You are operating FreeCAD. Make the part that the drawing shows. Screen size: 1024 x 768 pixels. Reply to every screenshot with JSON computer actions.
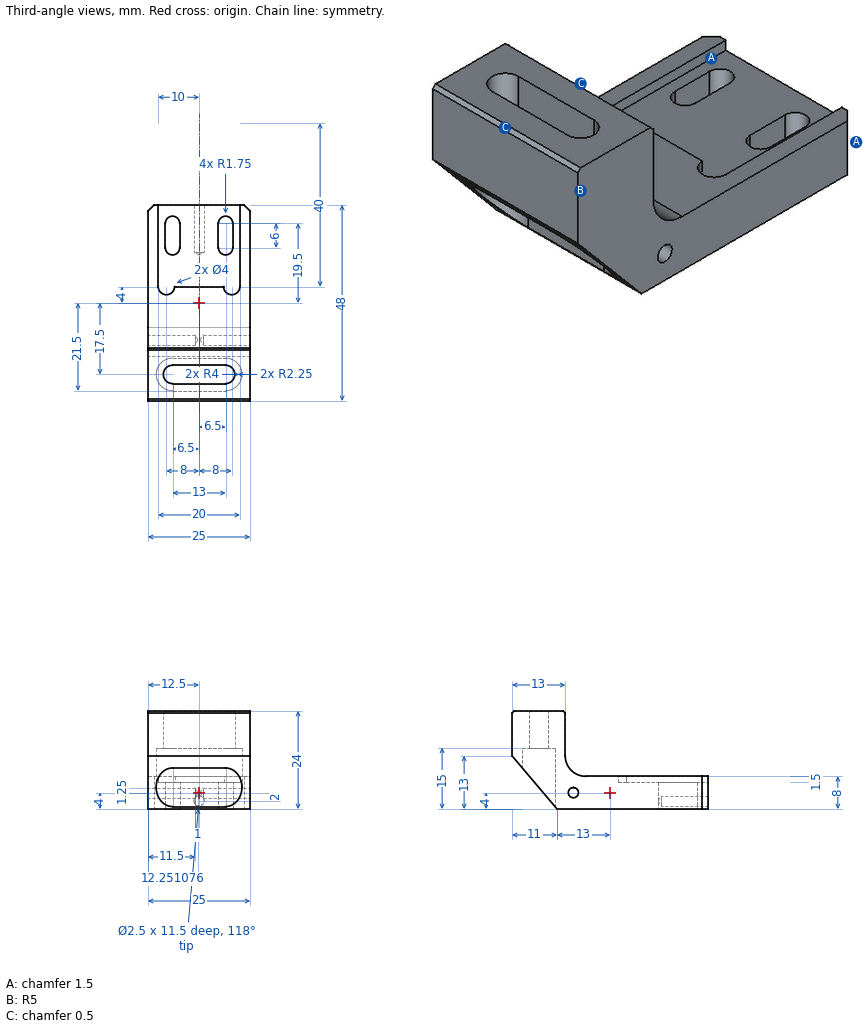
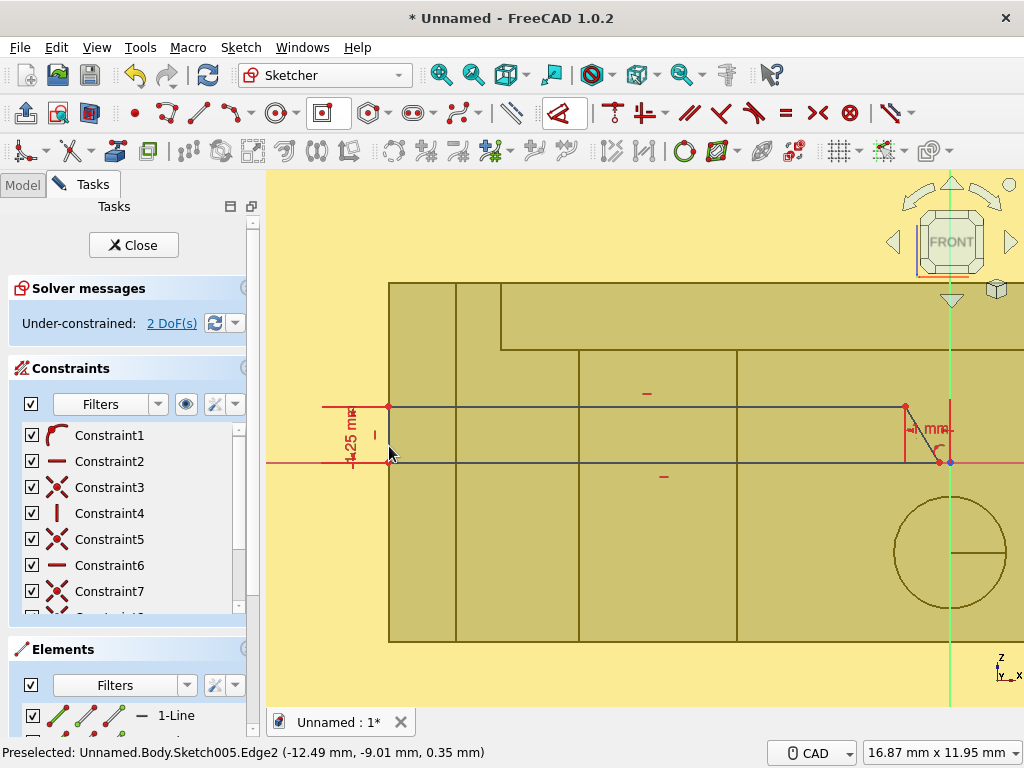
{"action": "left_click", "coordinate": [544, 407]}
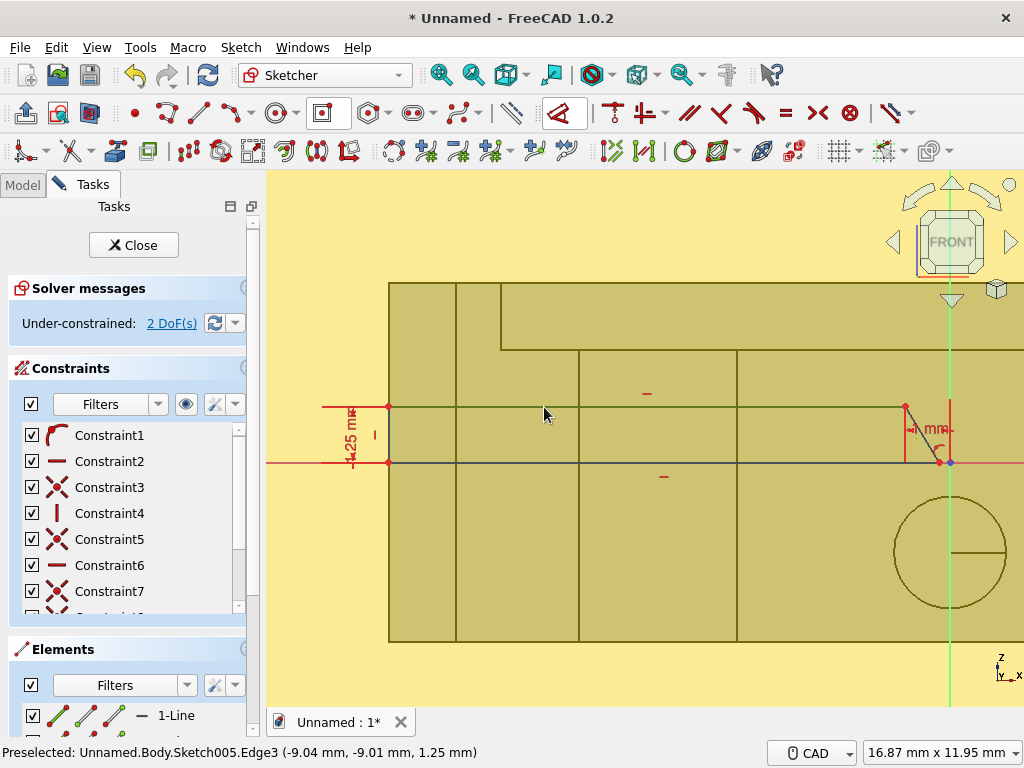
{"action": "left_click", "coordinate": [582, 114]}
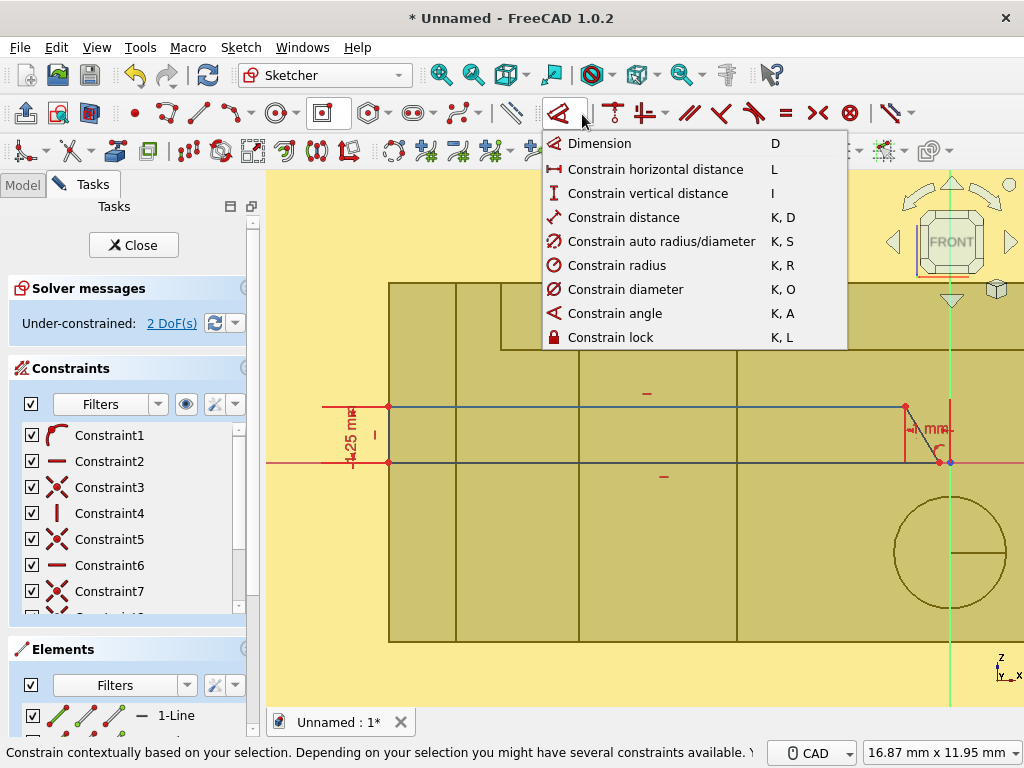
{"action": "left_click", "coordinate": [695, 169]}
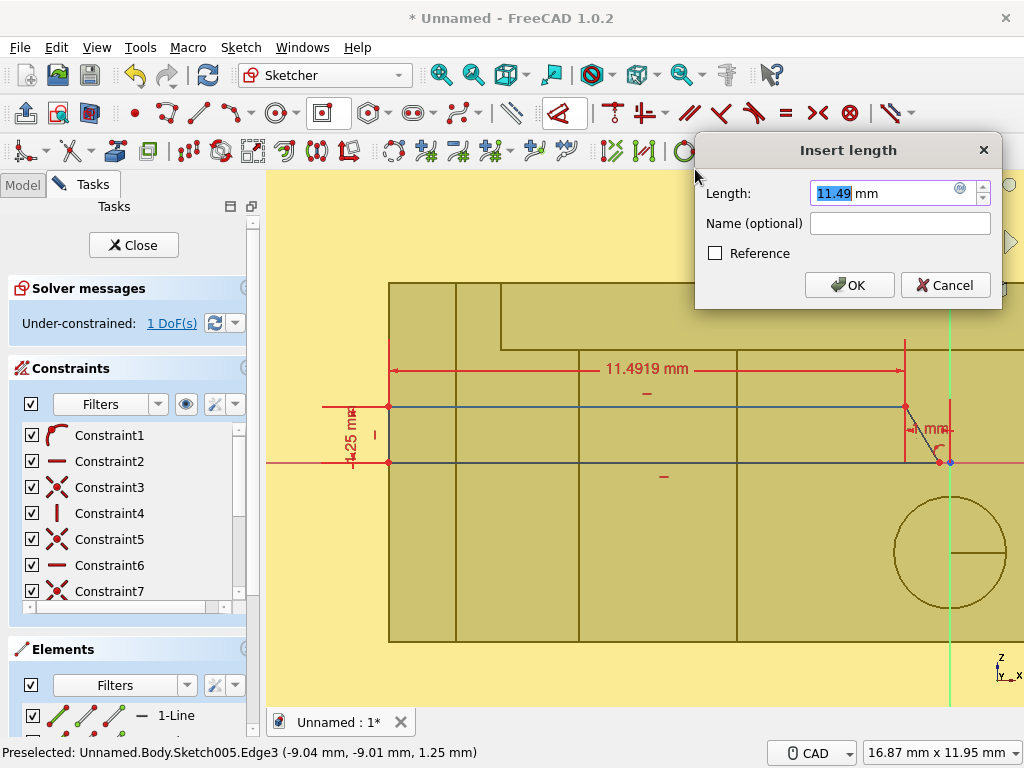
{"action": "type", "text": "11.5"}
{"action": "key", "text": "Return"}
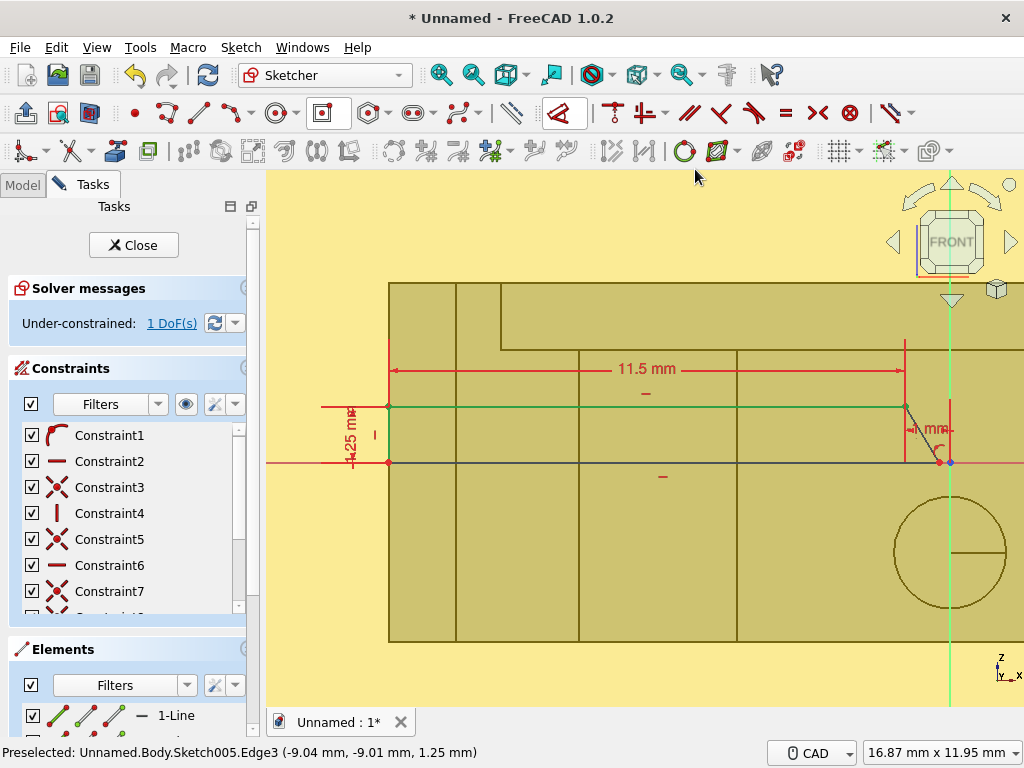
{"action": "left_click", "coordinate": [774, 463]}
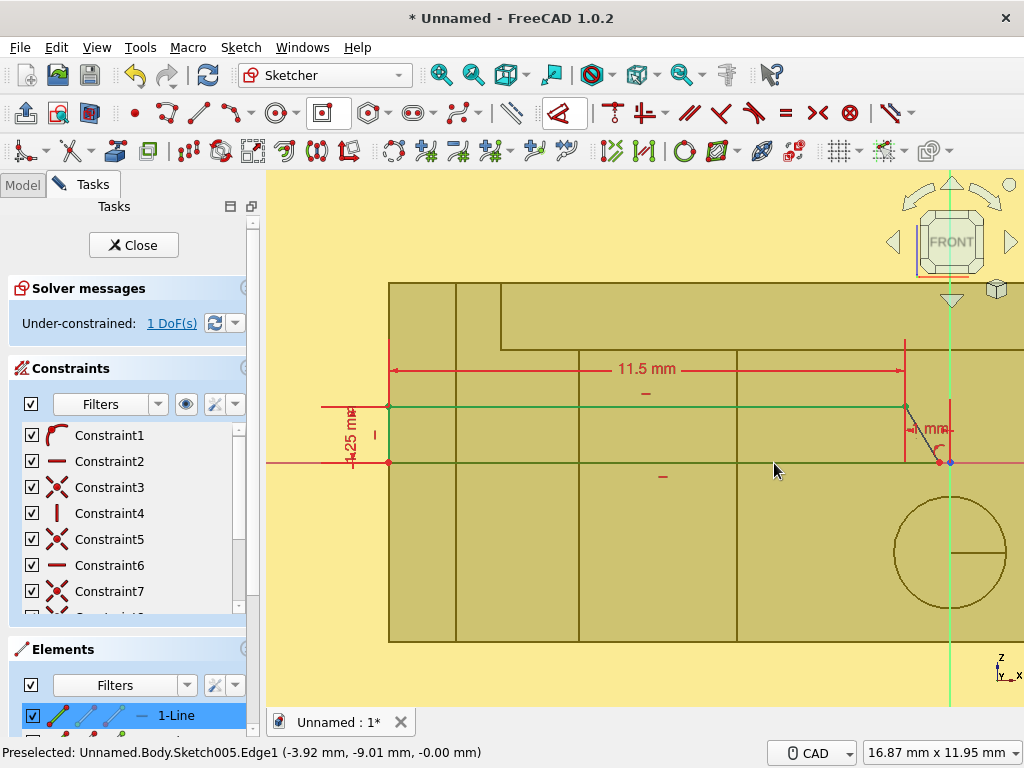
{"action": "left_click", "coordinate": [582, 114]}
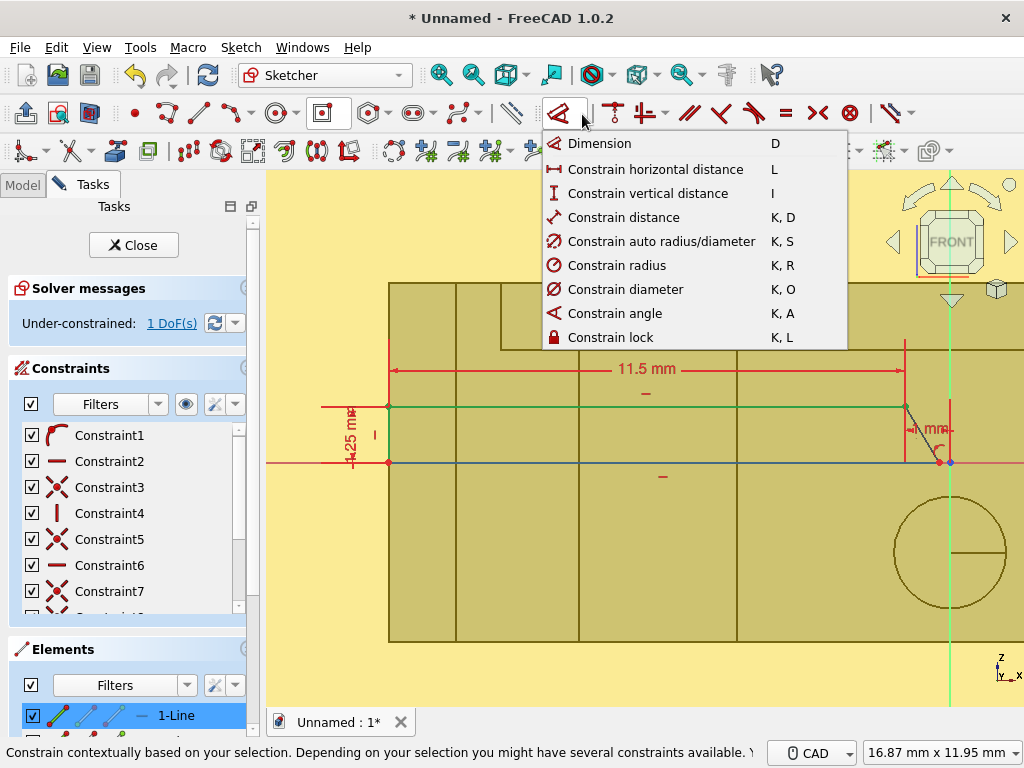
{"action": "left_click", "coordinate": [695, 169]}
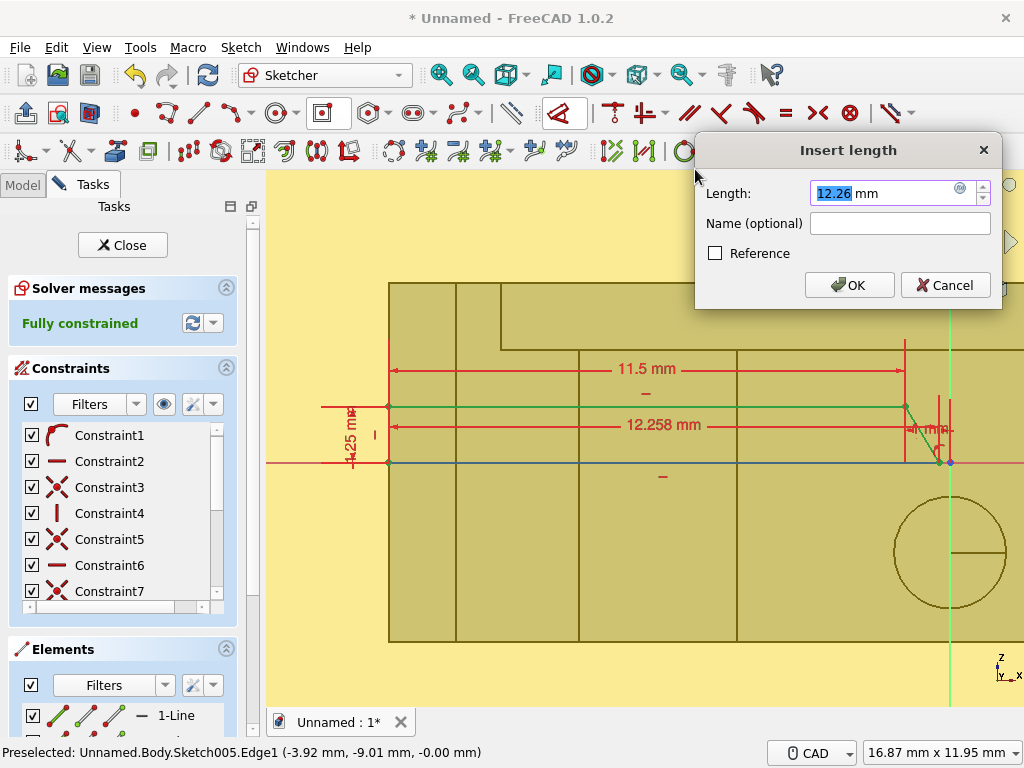
{"action": "type", "text": "12.251076"}
{"action": "key", "text": "Return"}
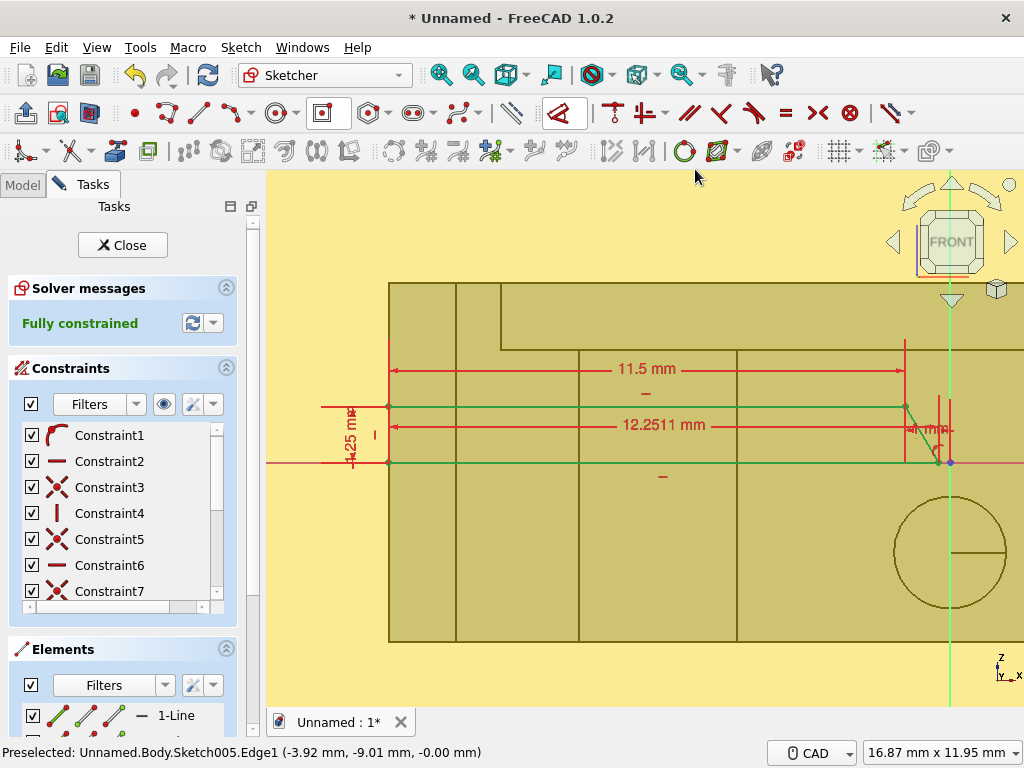
{"action": "left_click", "coordinate": [123, 245]}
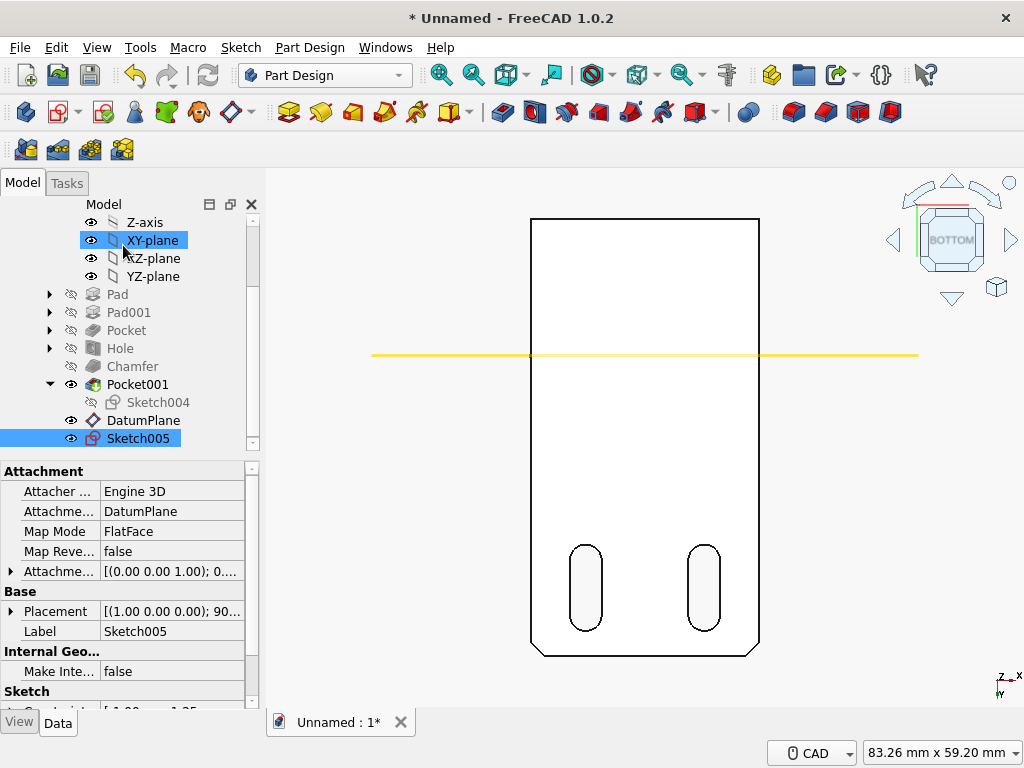
{"action": "left_click", "coordinate": [568, 112]}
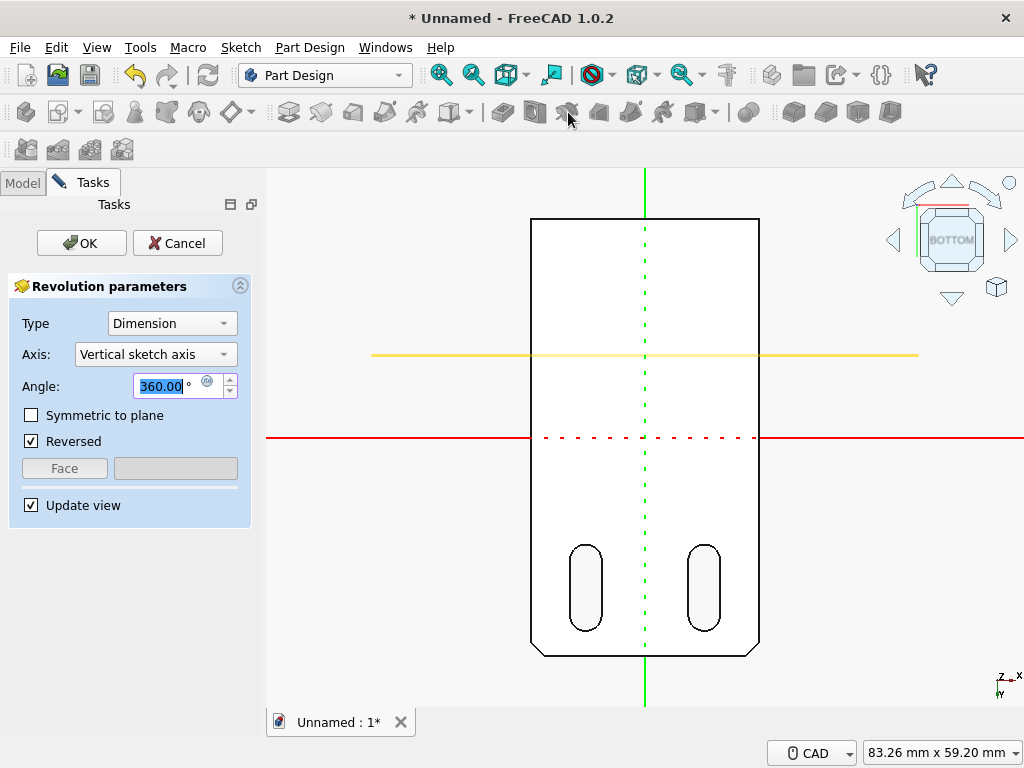
{"action": "left_click", "coordinate": [156, 354]}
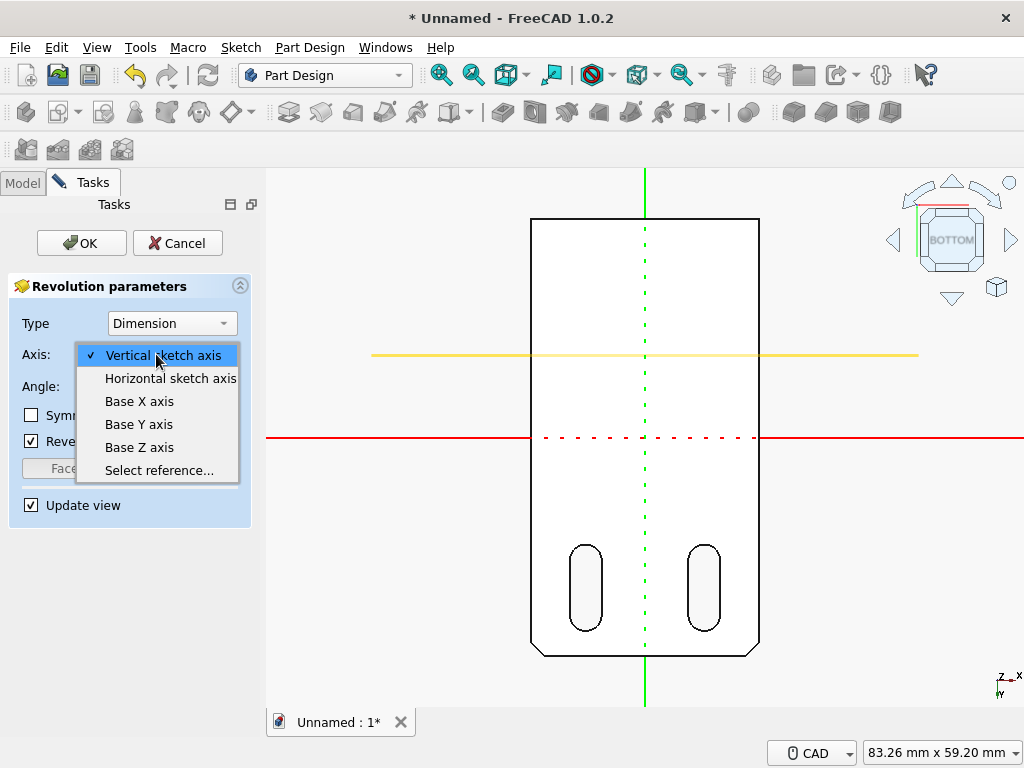
{"action": "left_click", "coordinate": [156, 378]}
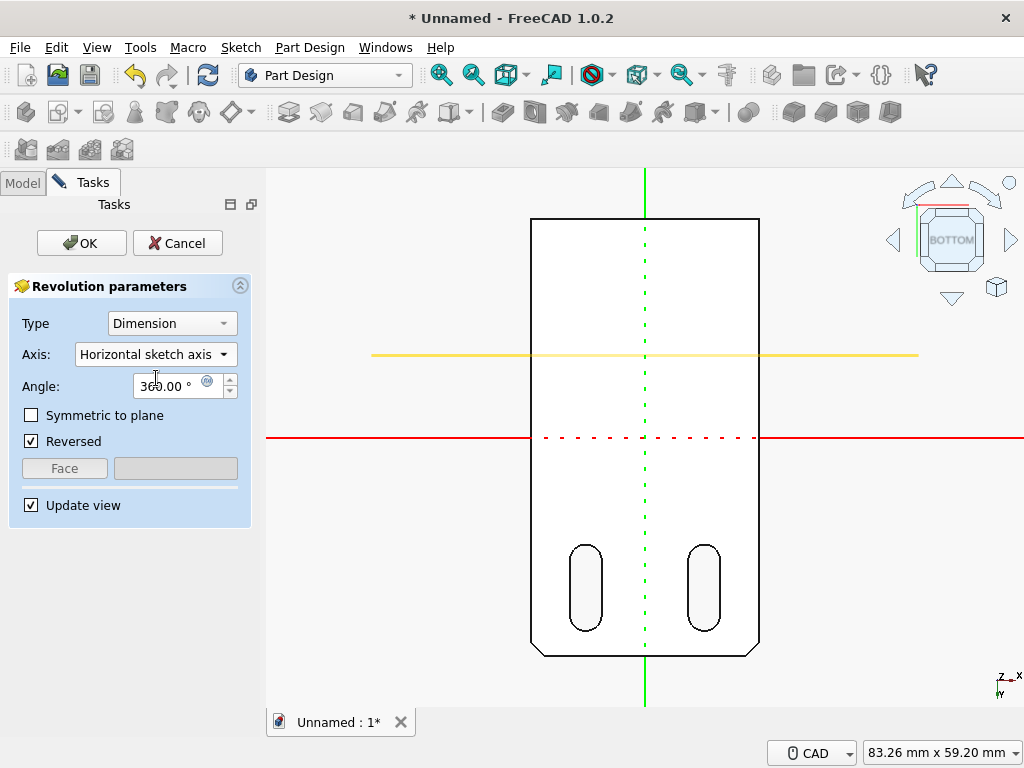
{"action": "left_click", "coordinate": [82, 243]}